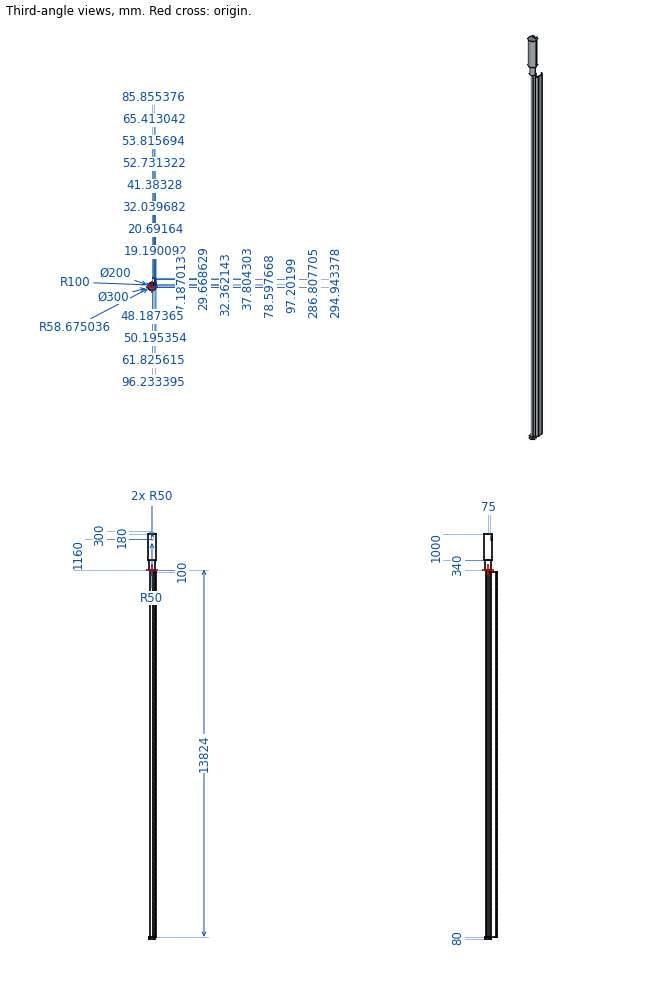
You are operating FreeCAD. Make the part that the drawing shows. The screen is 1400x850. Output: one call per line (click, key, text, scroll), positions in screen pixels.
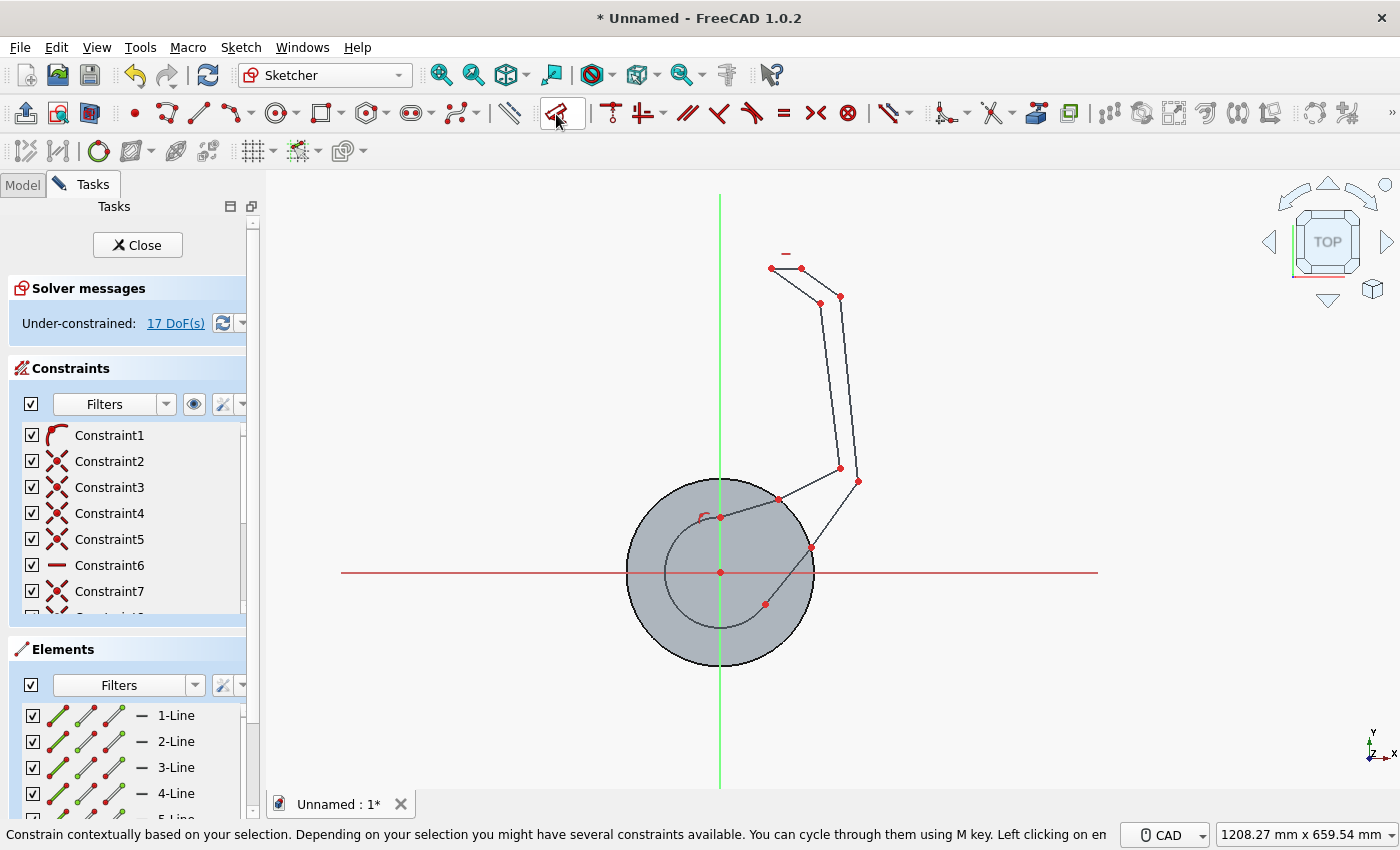
click(668, 554)
click(638, 543)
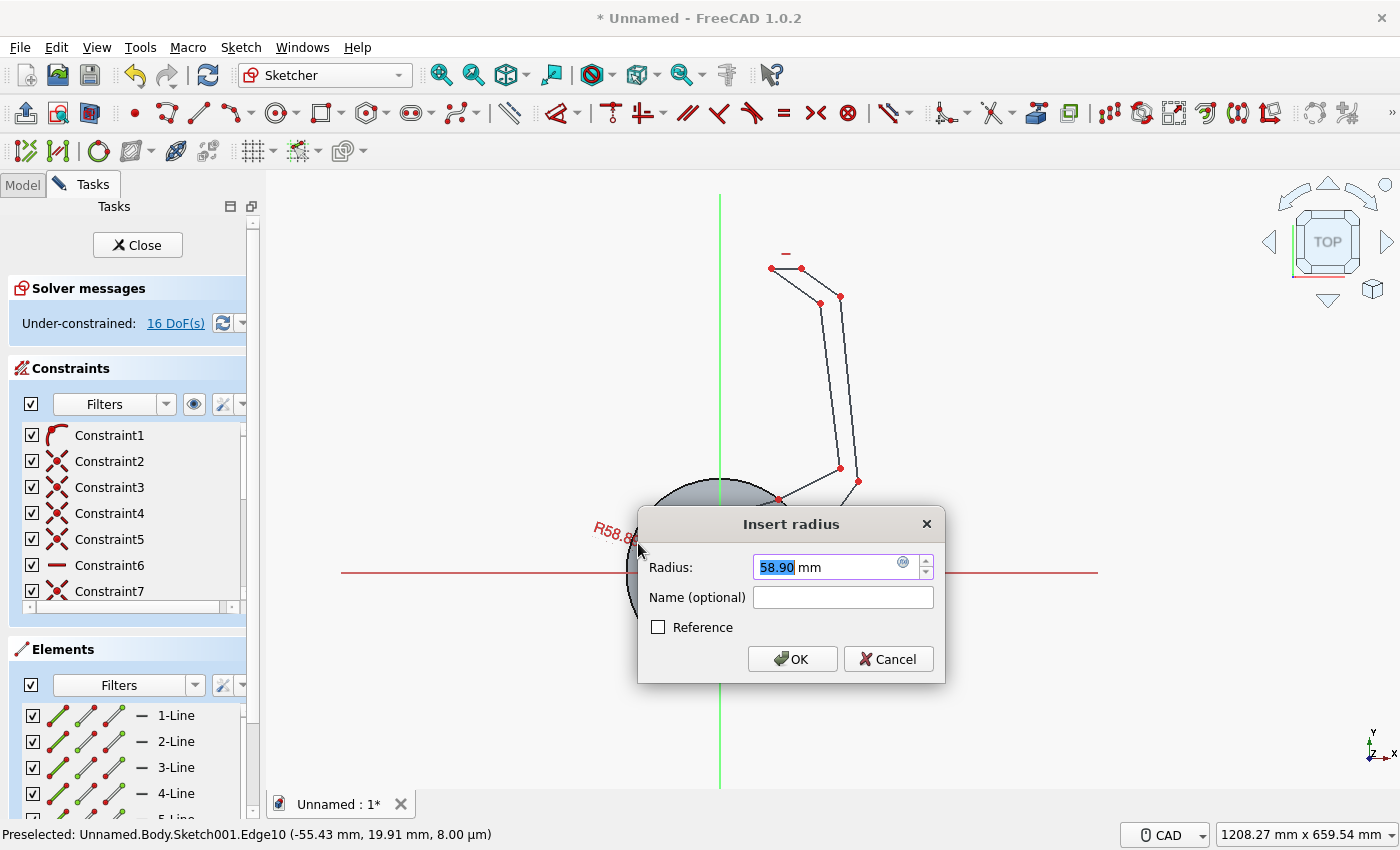
text(58.675036)
key(Return)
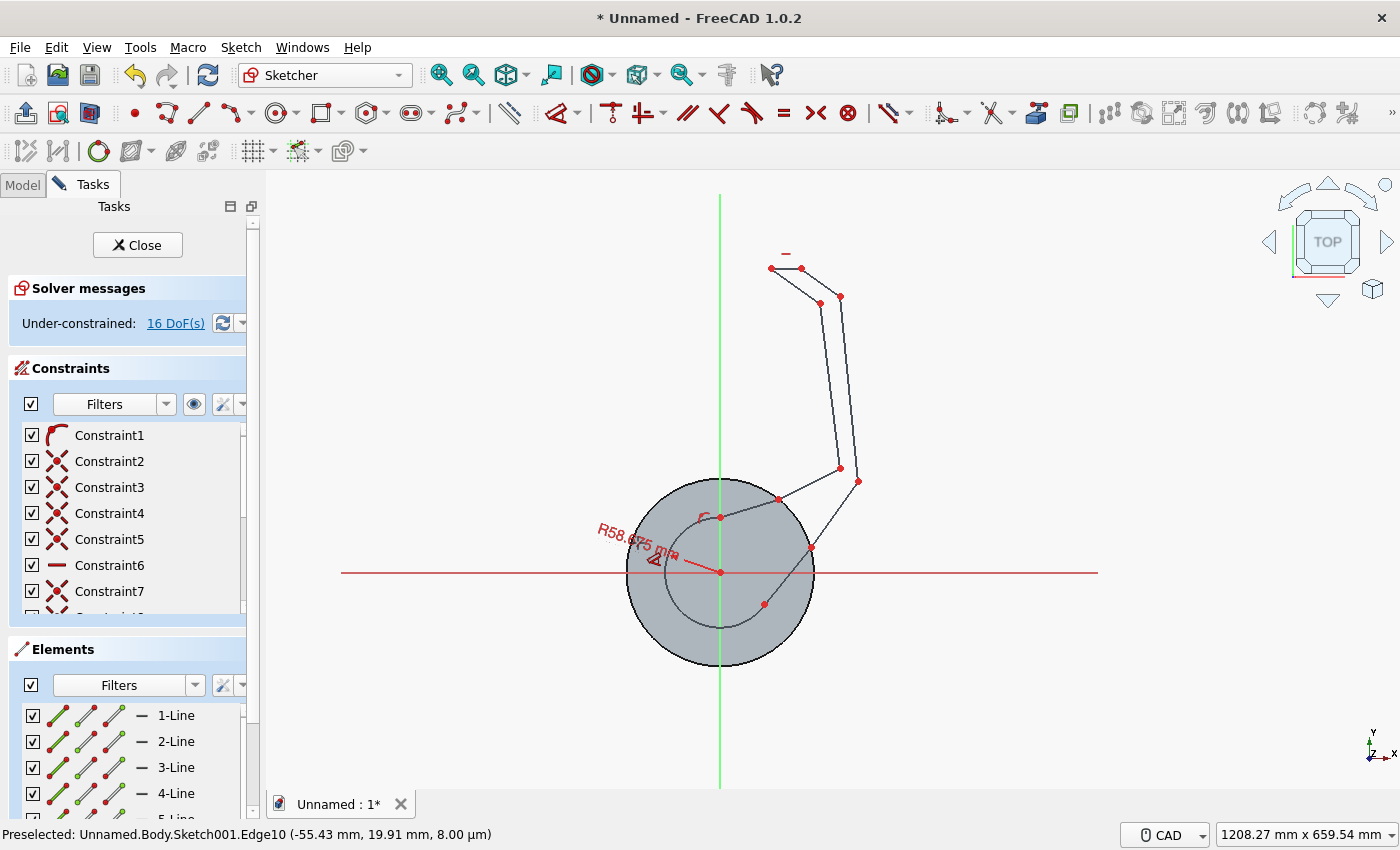
scroll(792, 269, up, 3)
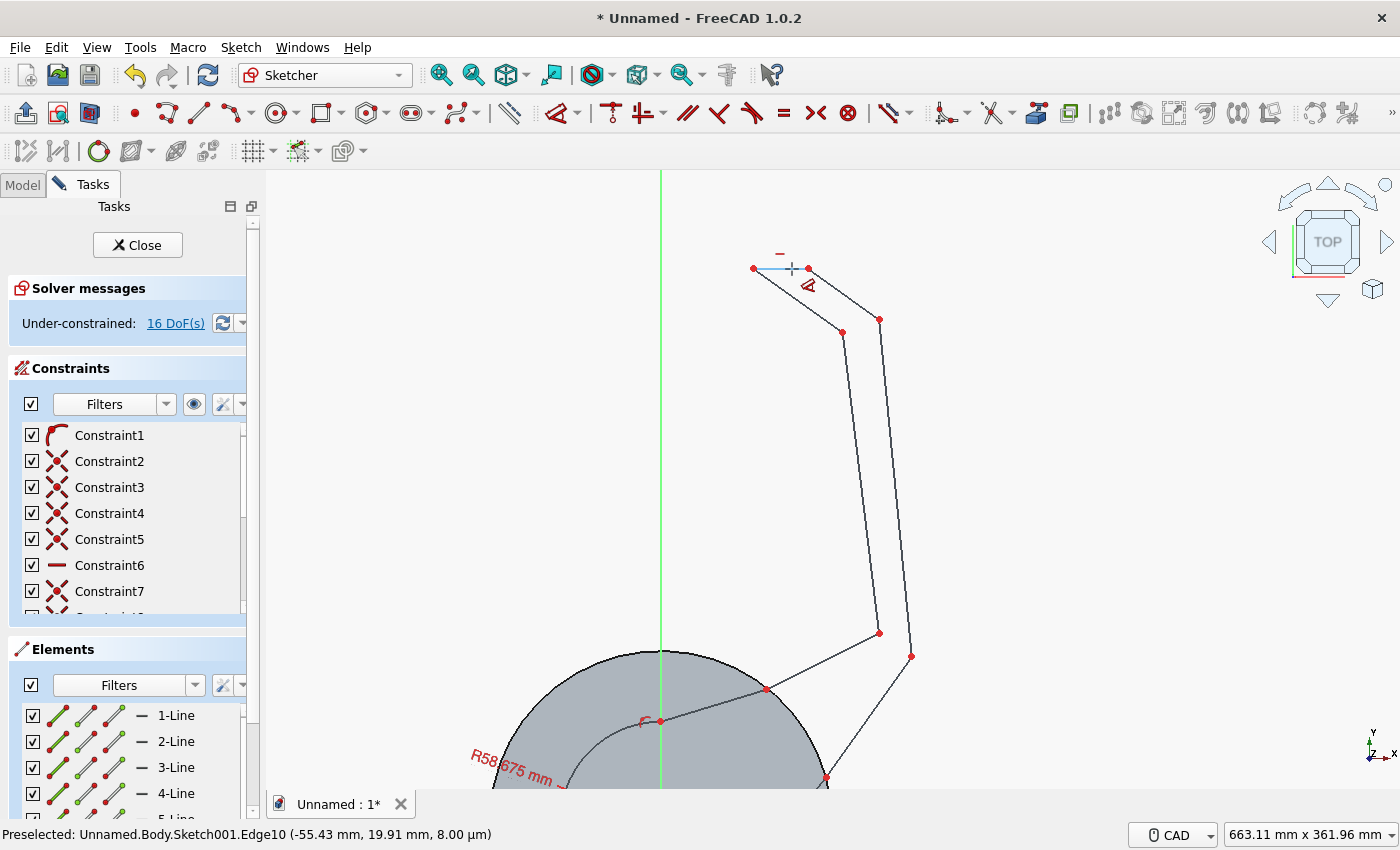
click(792, 269)
click(781, 235)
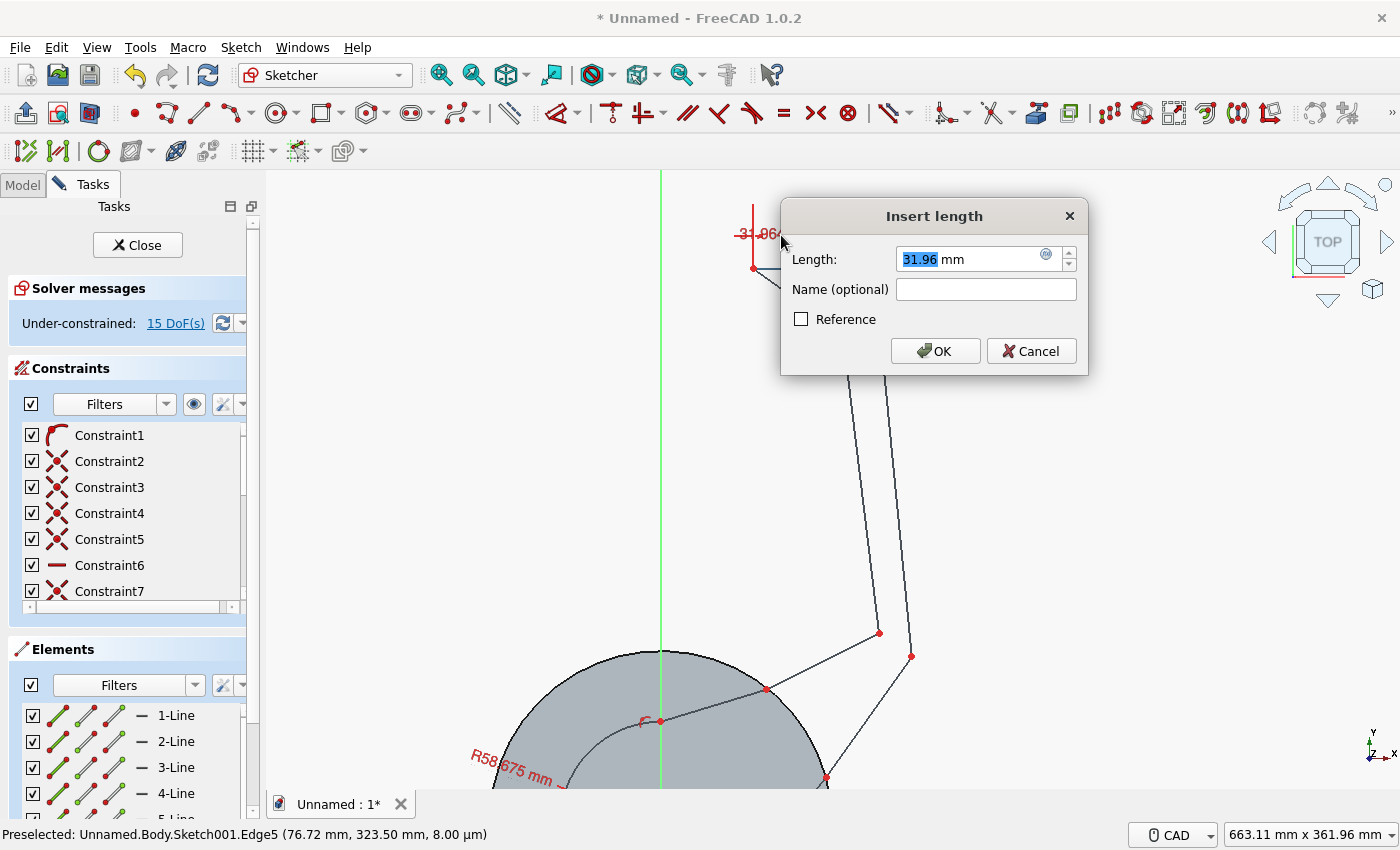
text(32.039682)
key(Return)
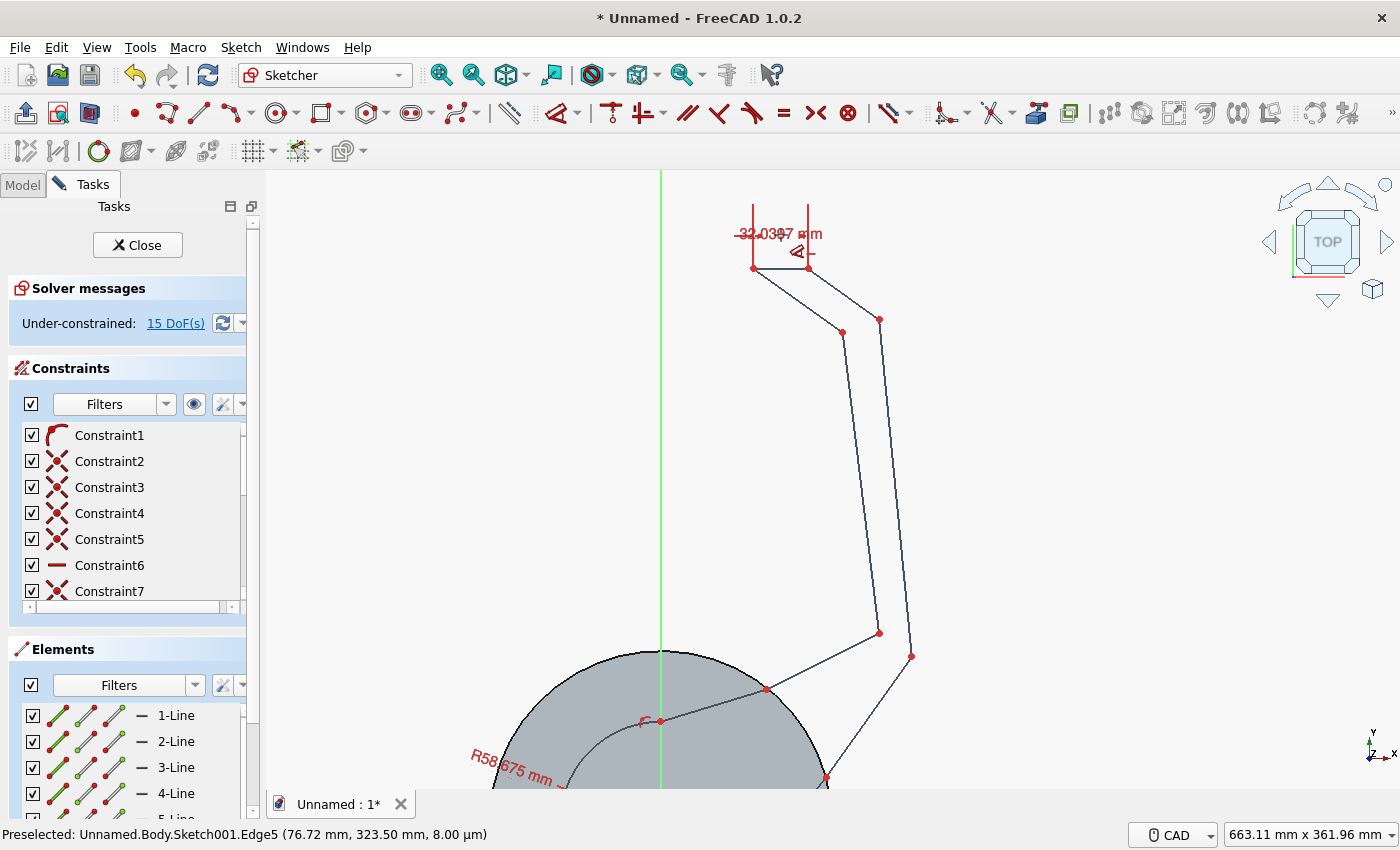
click(912, 657)
click(946, 709)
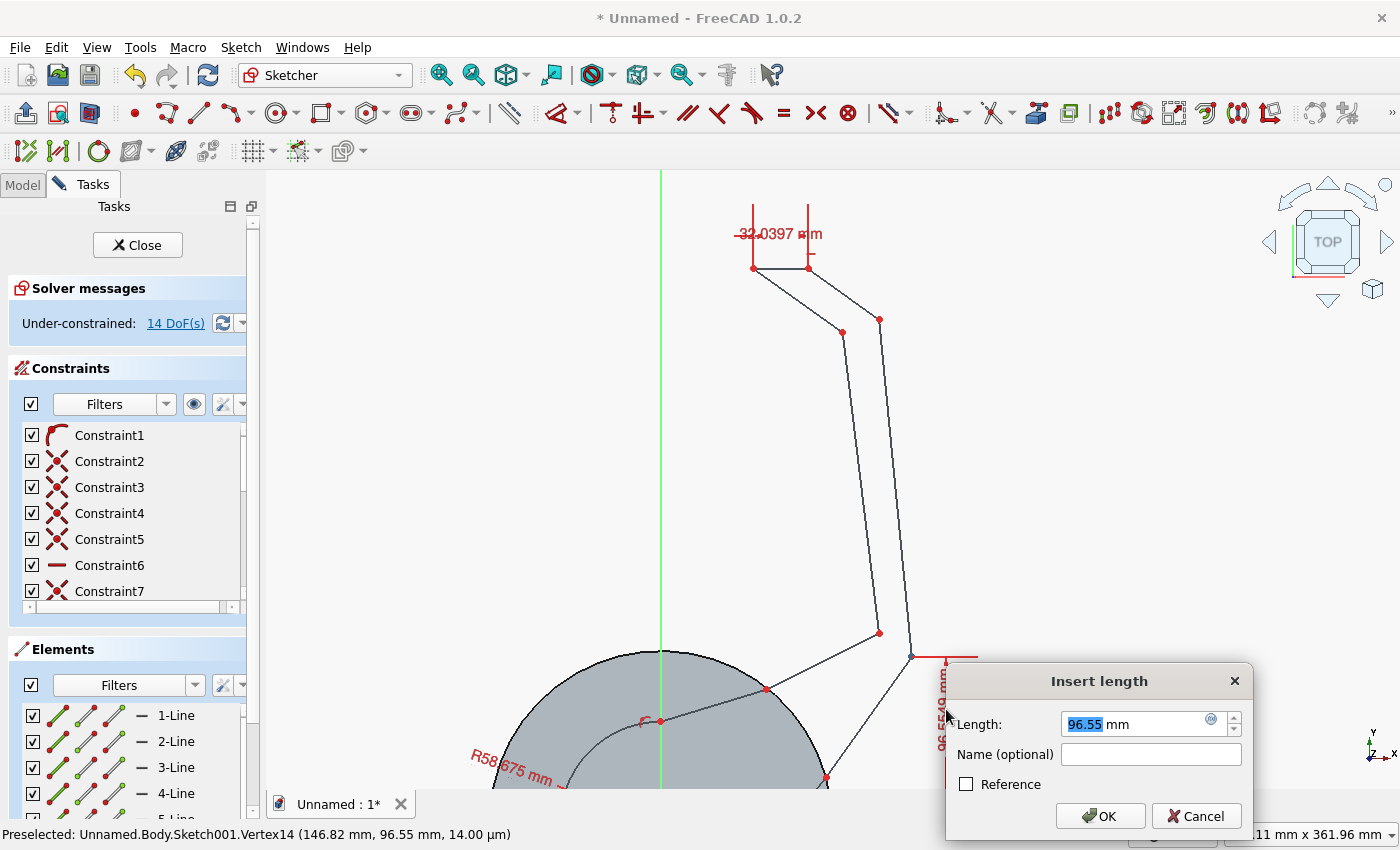
text(97.20199)
key(Return)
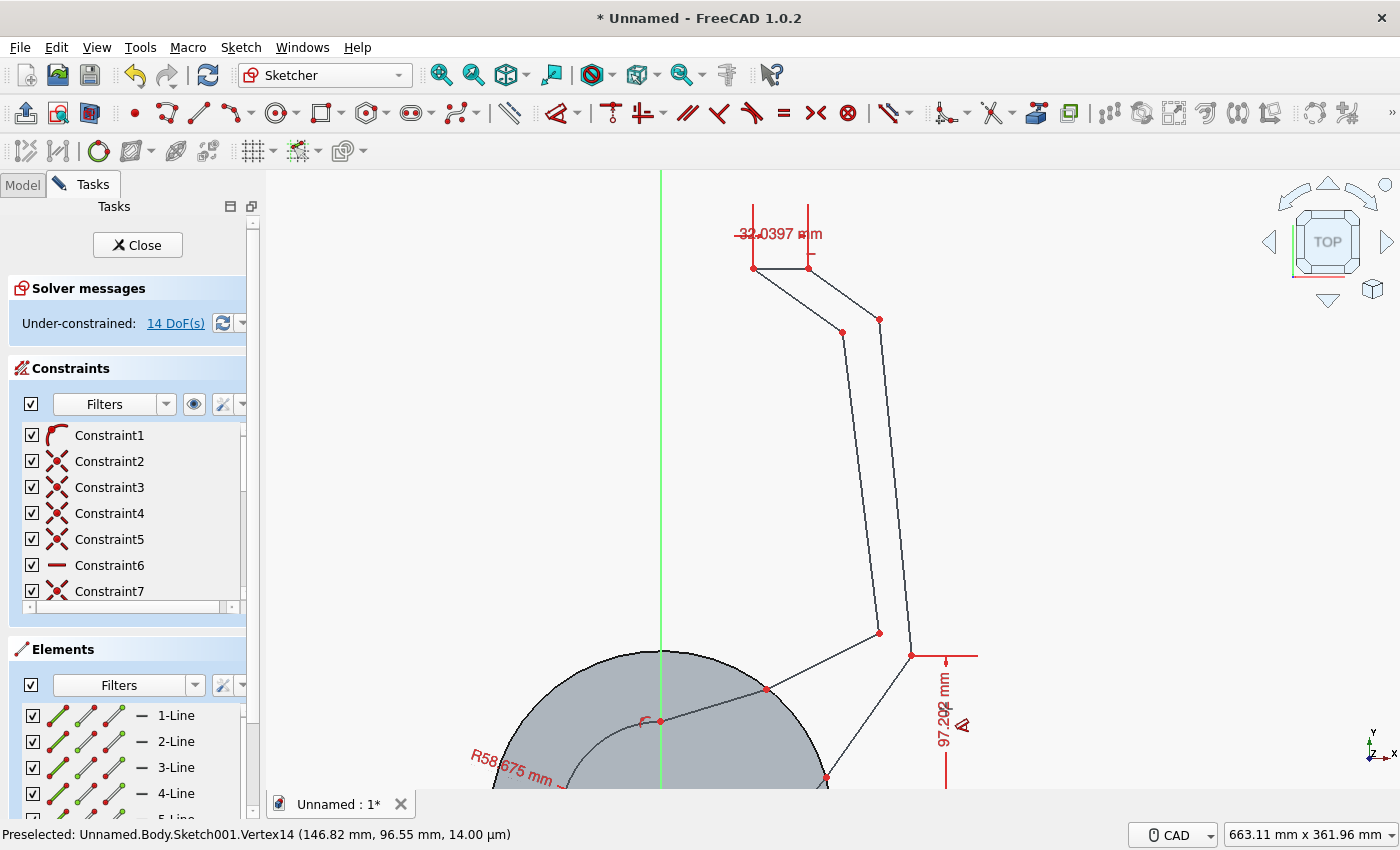
click(868, 543)
click(874, 299)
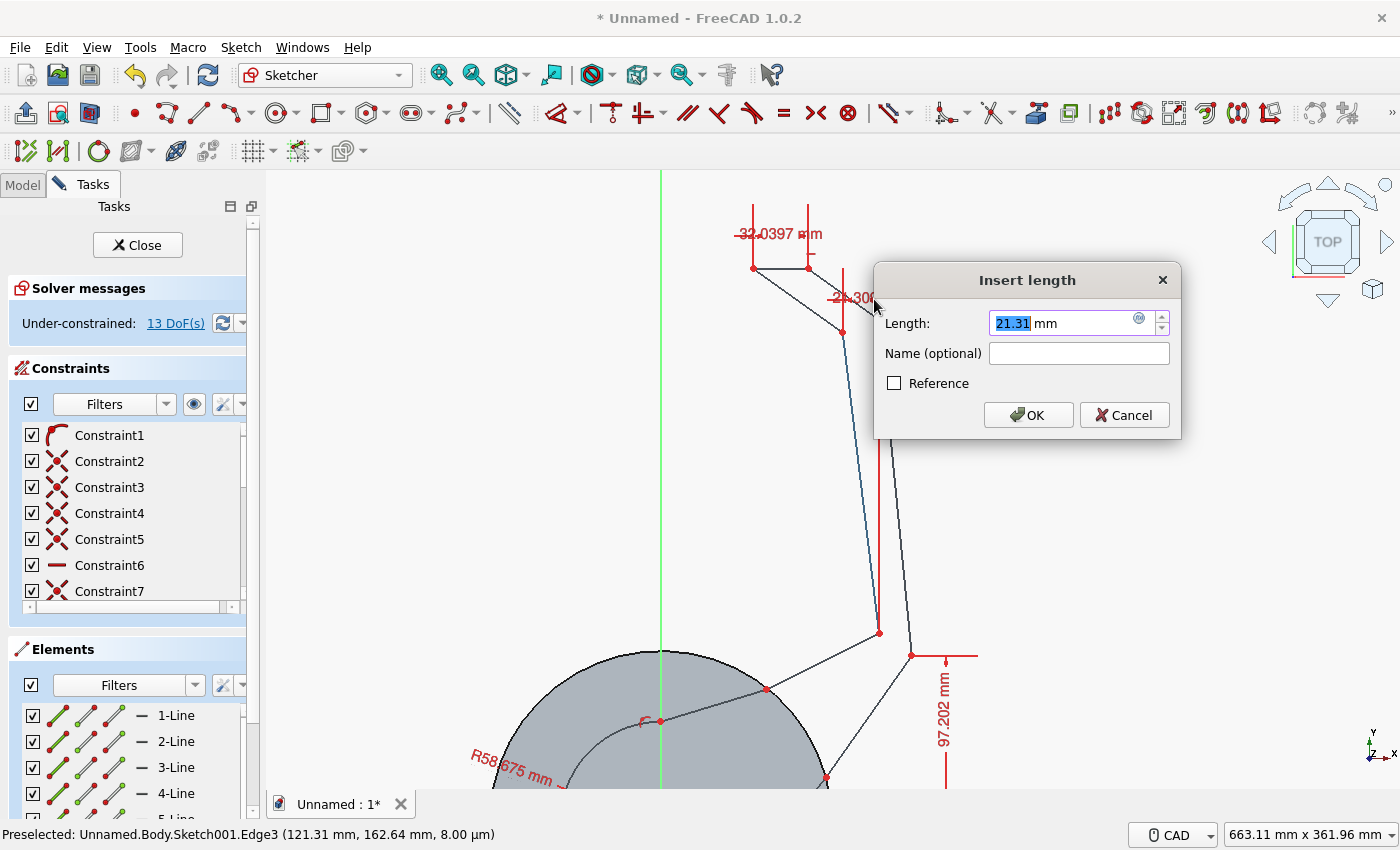
text(20.69164)
key(Return)